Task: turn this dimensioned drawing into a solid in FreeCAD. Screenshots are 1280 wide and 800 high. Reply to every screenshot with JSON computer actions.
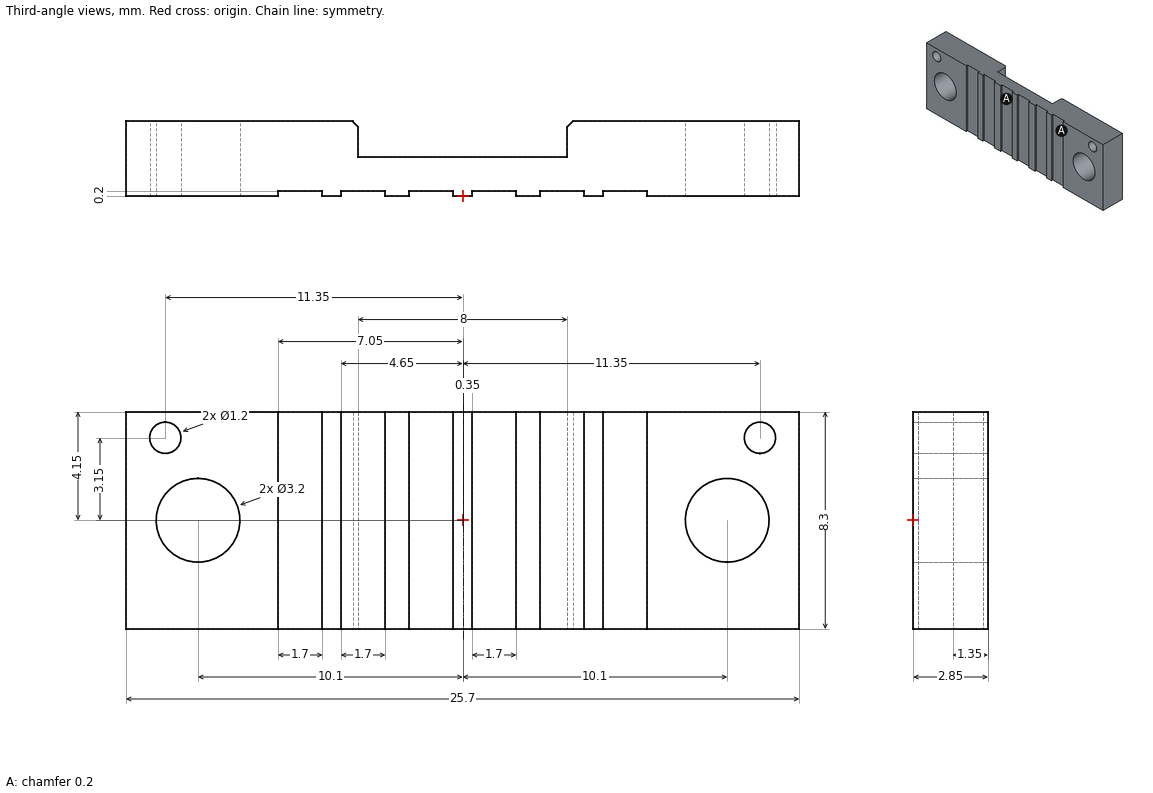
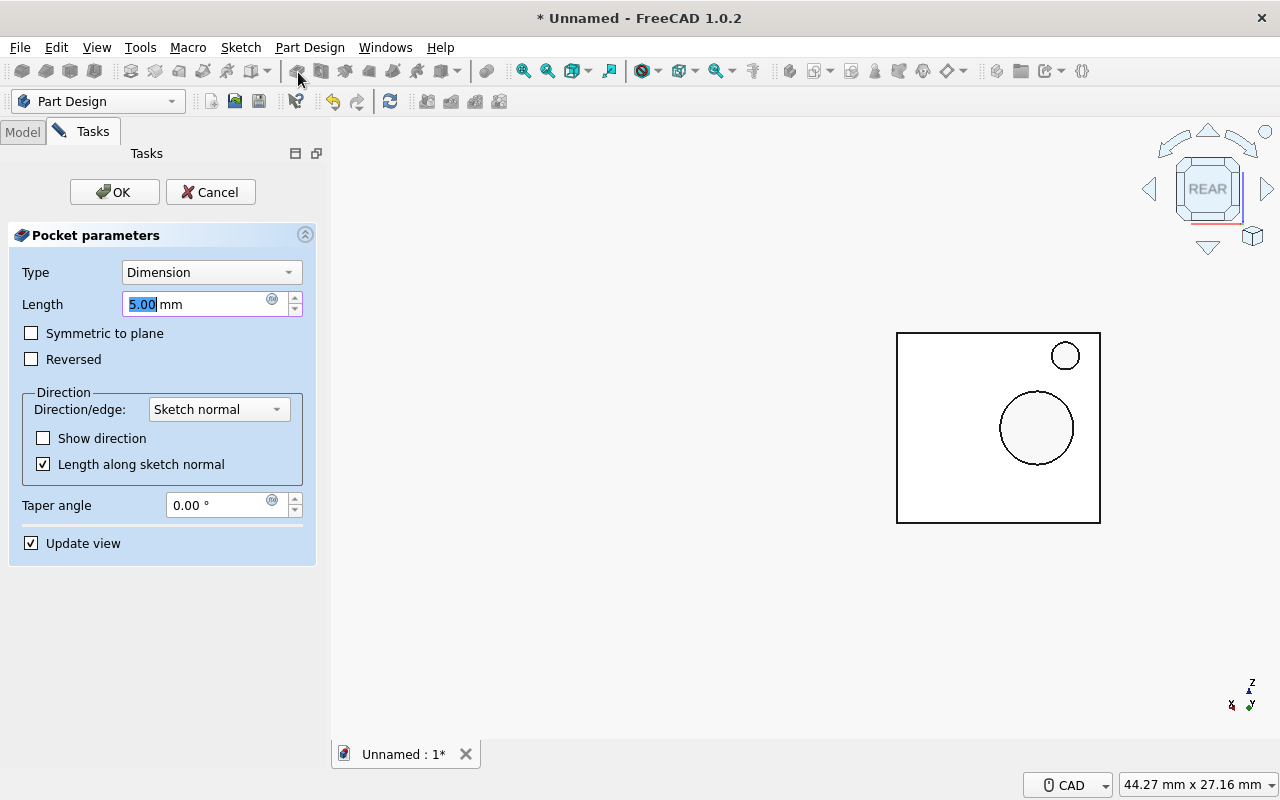
{"action": "type", "text": "1.35"}
{"action": "key", "text": "Tab"}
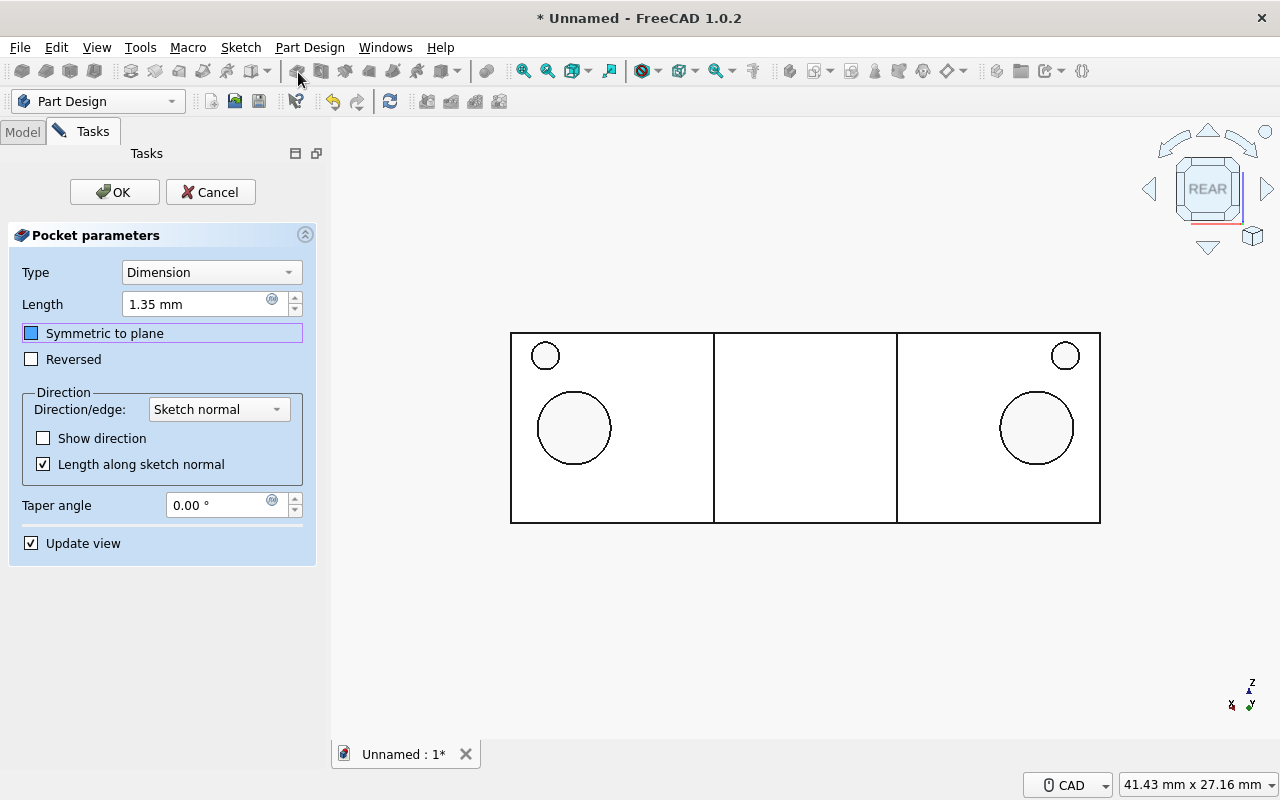
{"action": "left_click", "coordinate": [115, 192]}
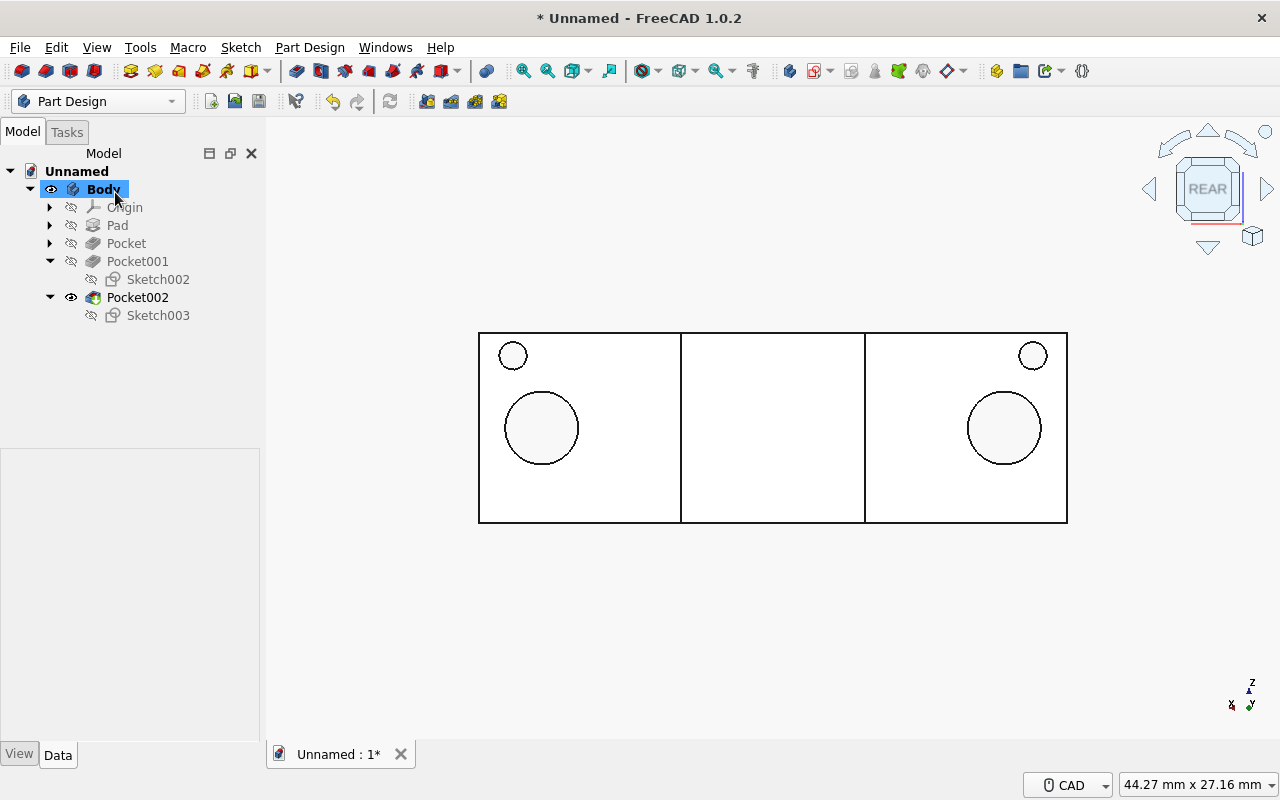
{"action": "left_click", "coordinate": [681, 427]}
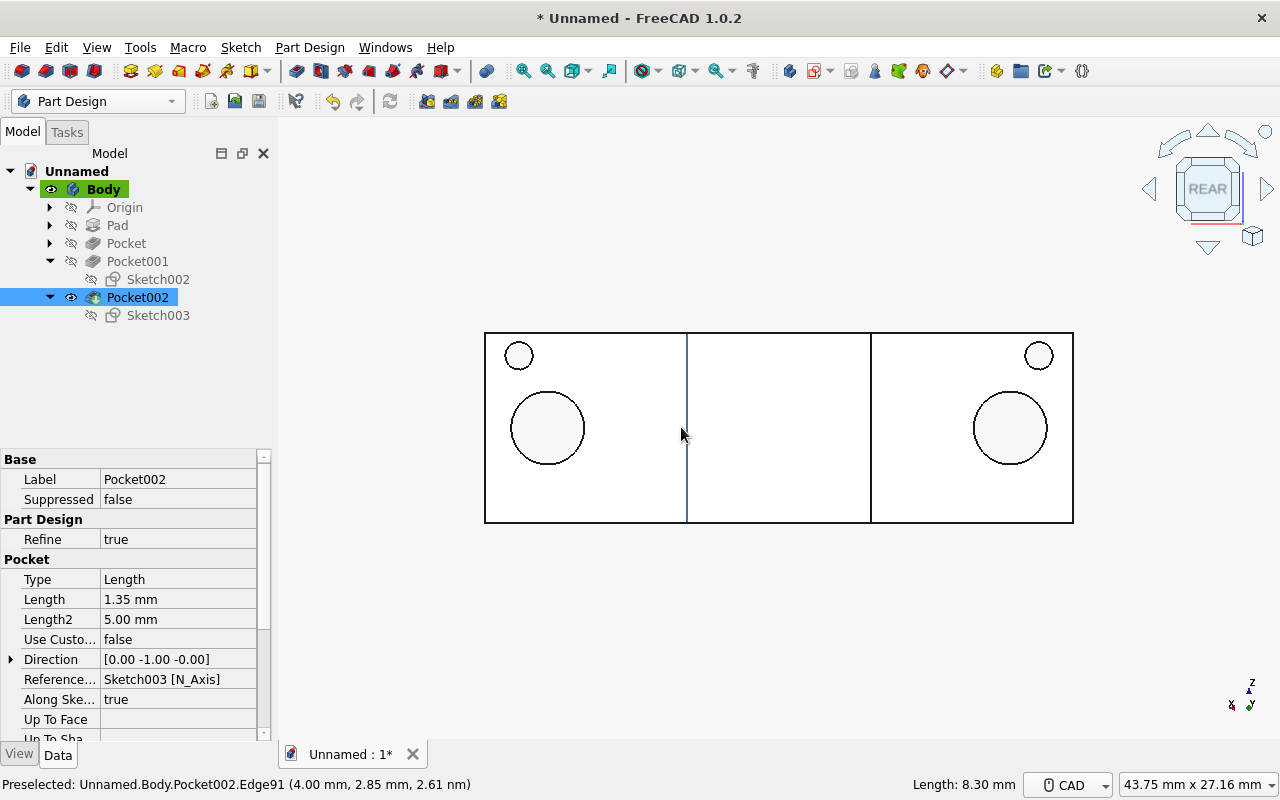
{"action": "key", "text": "0"}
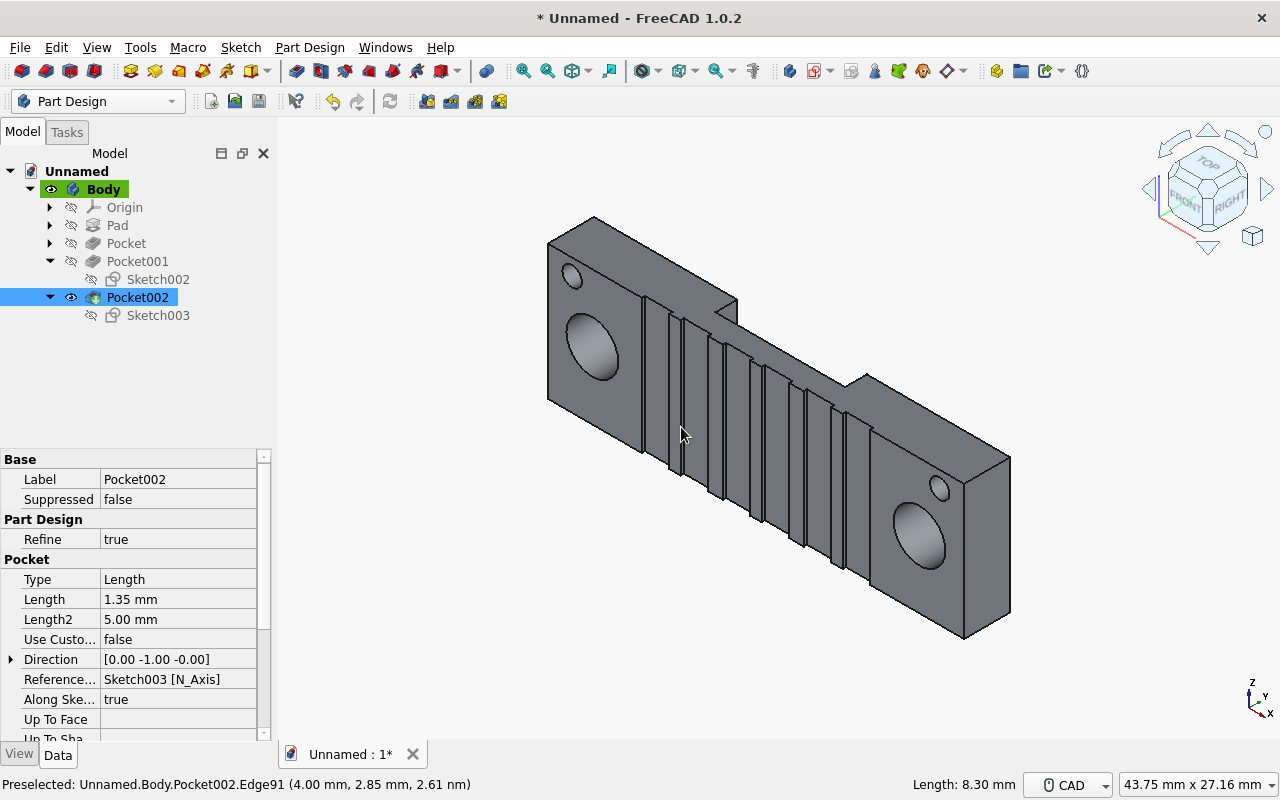
{"action": "key", "text": "2"}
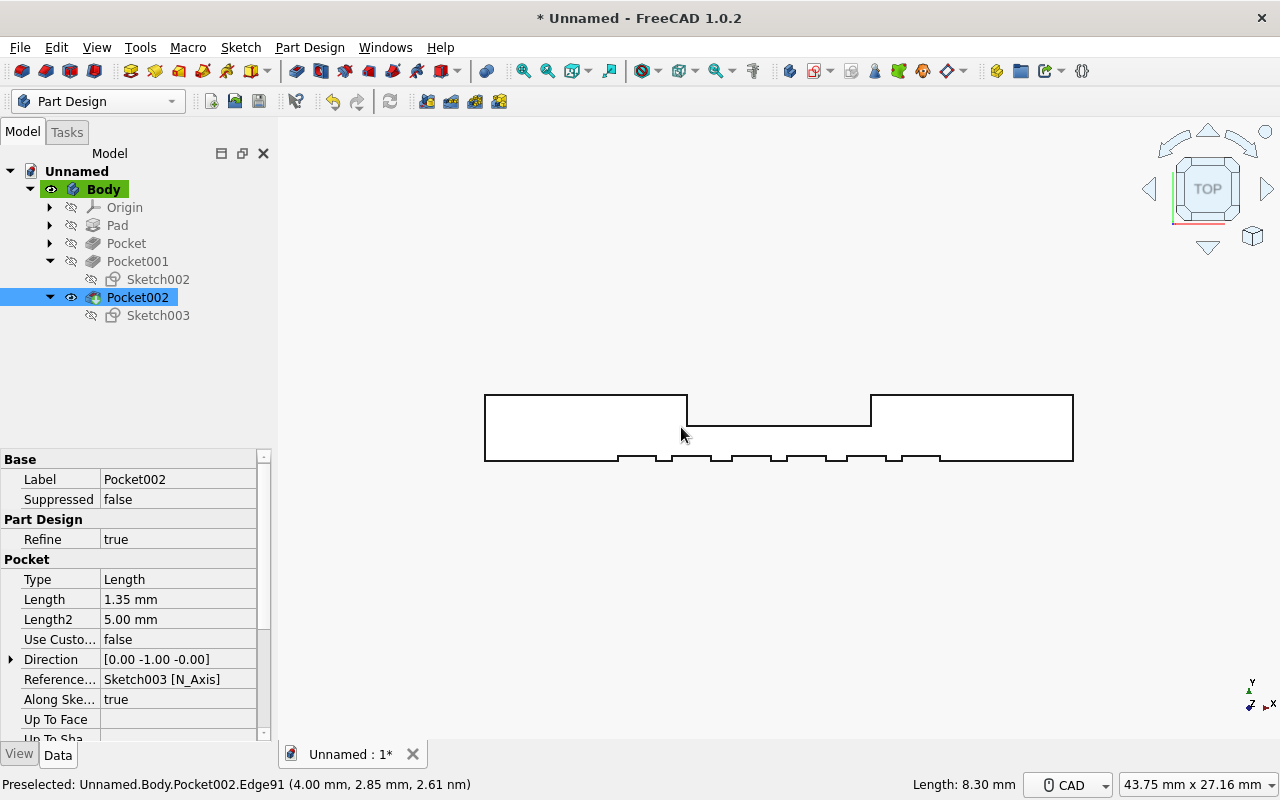
{"action": "key", "text": "1"}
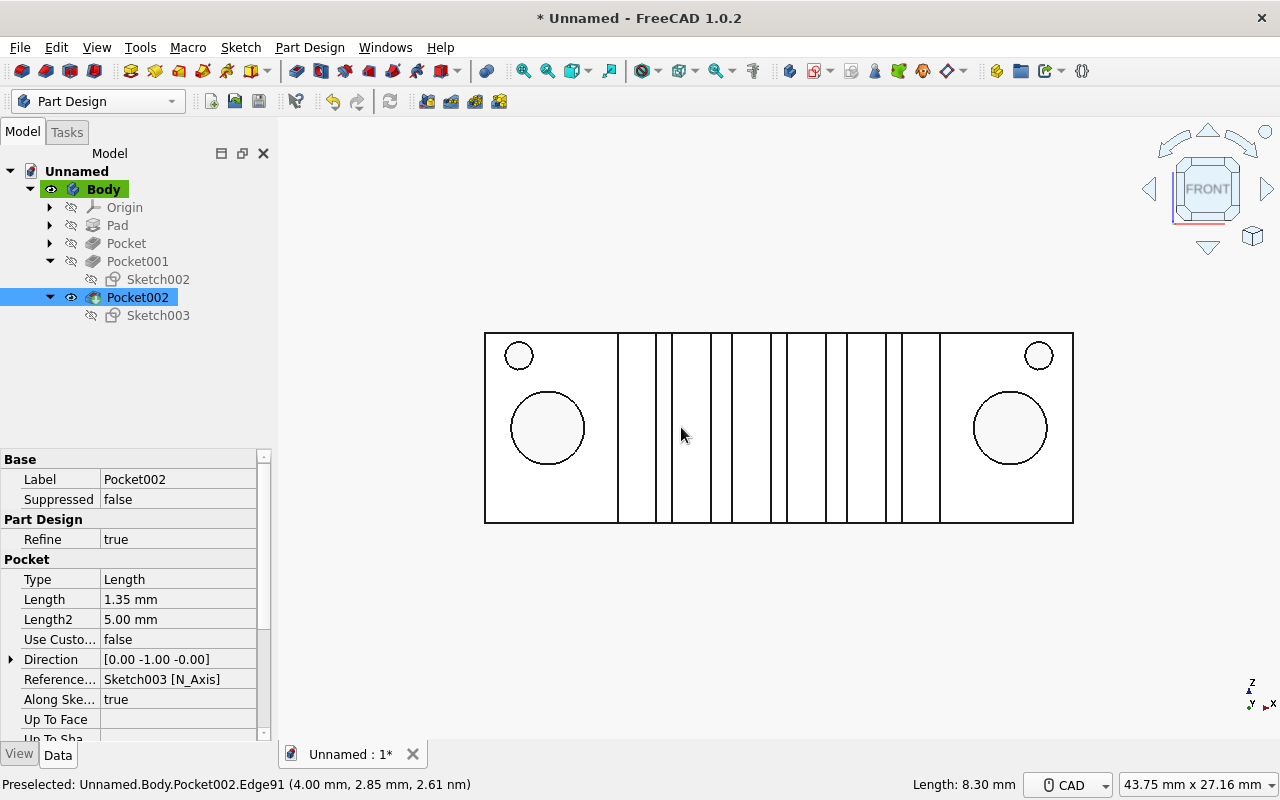
{"action": "key", "text": "3"}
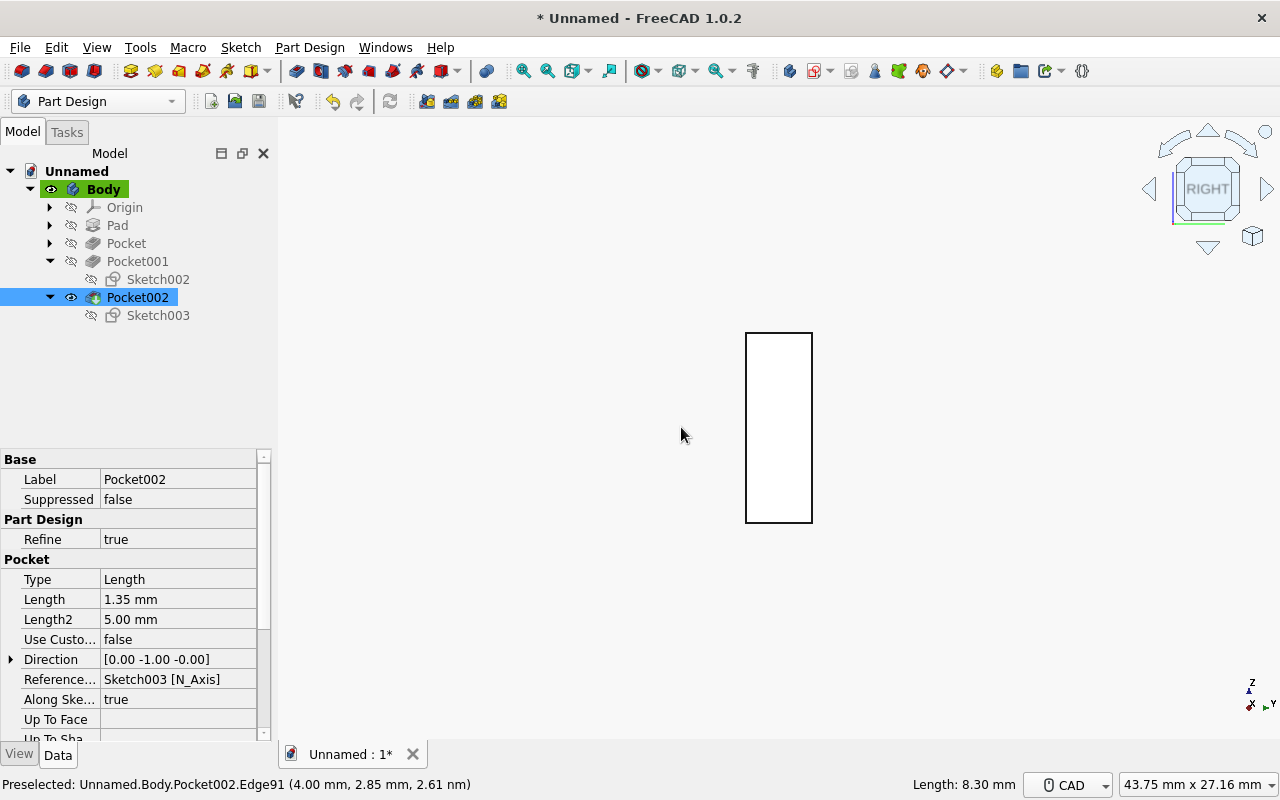
{"action": "left_click", "coordinate": [524, 72]}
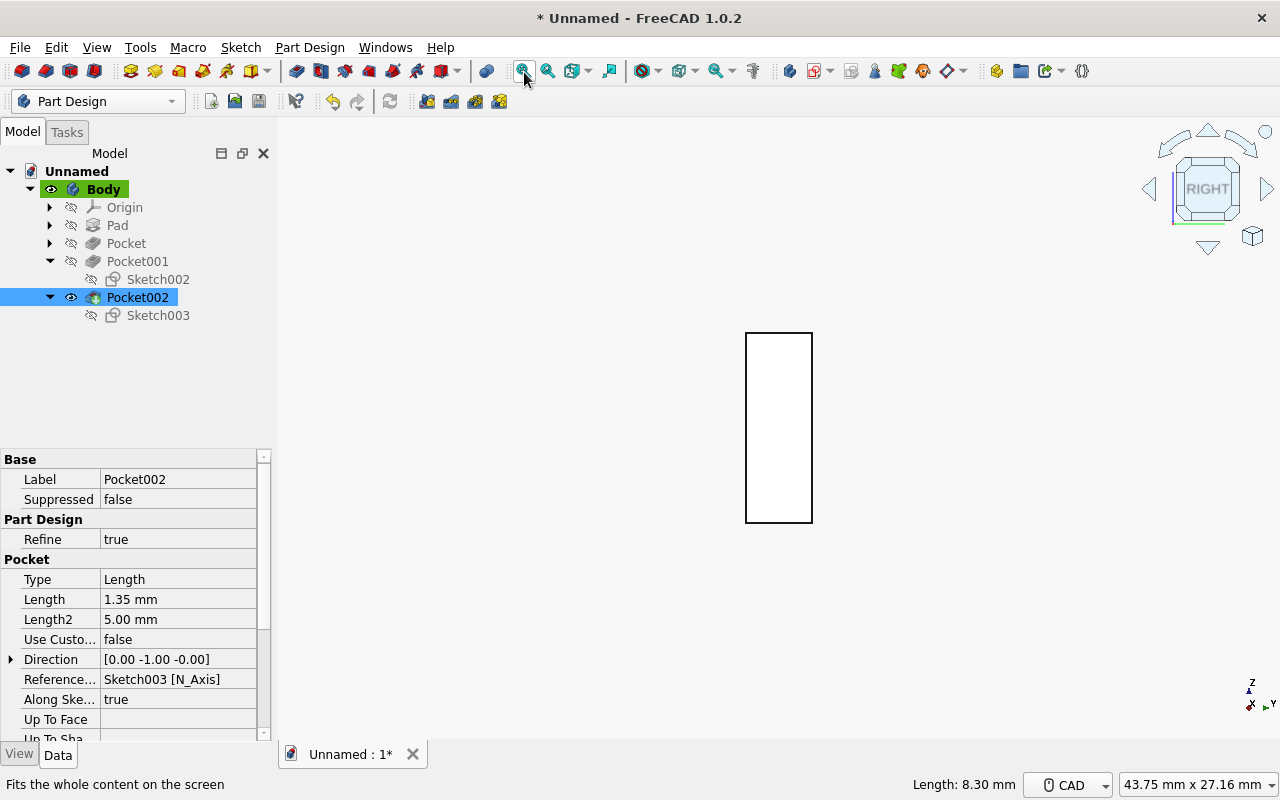
{"action": "key", "text": "5"}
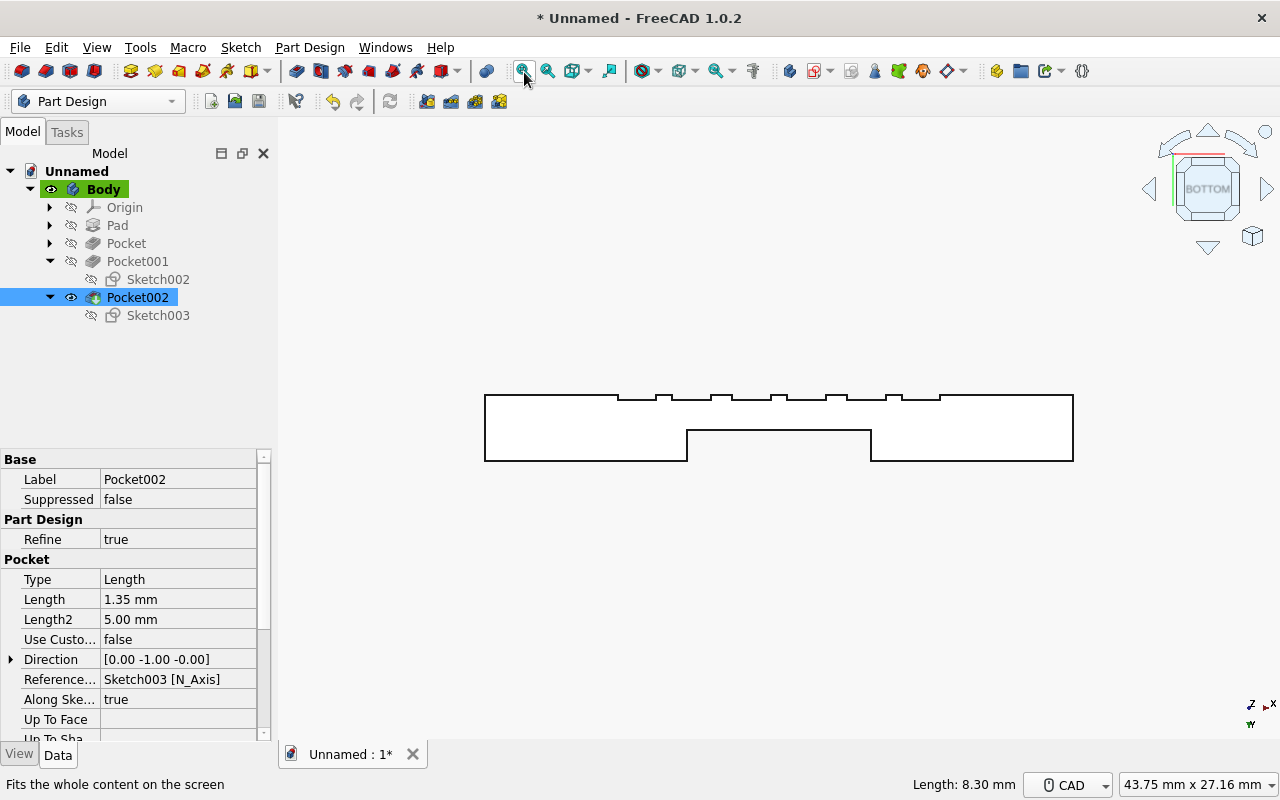
{"action": "key", "text": "4"}